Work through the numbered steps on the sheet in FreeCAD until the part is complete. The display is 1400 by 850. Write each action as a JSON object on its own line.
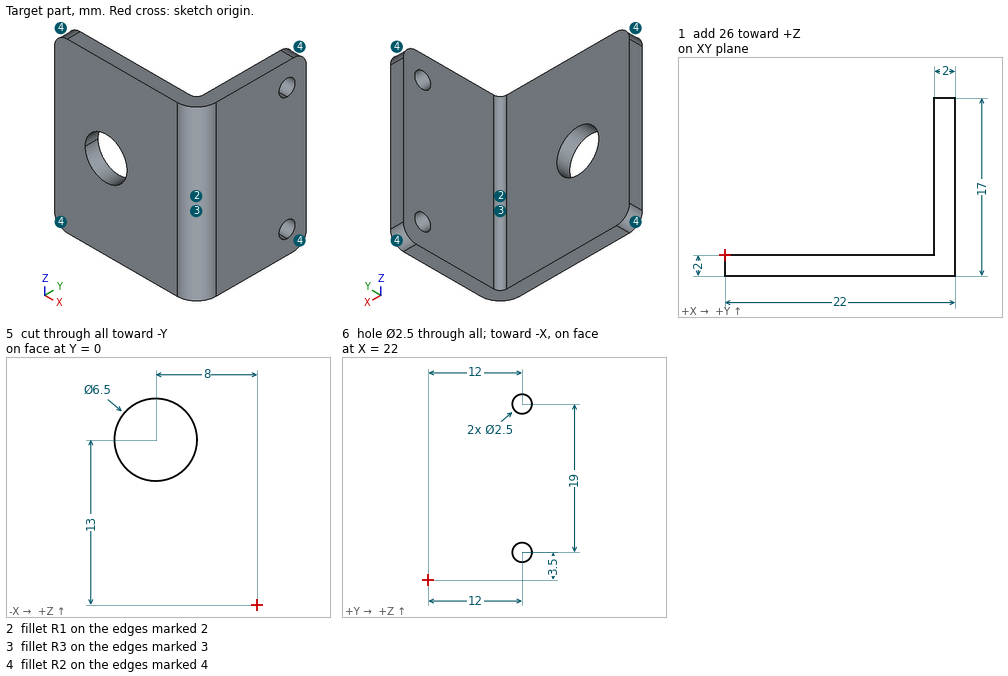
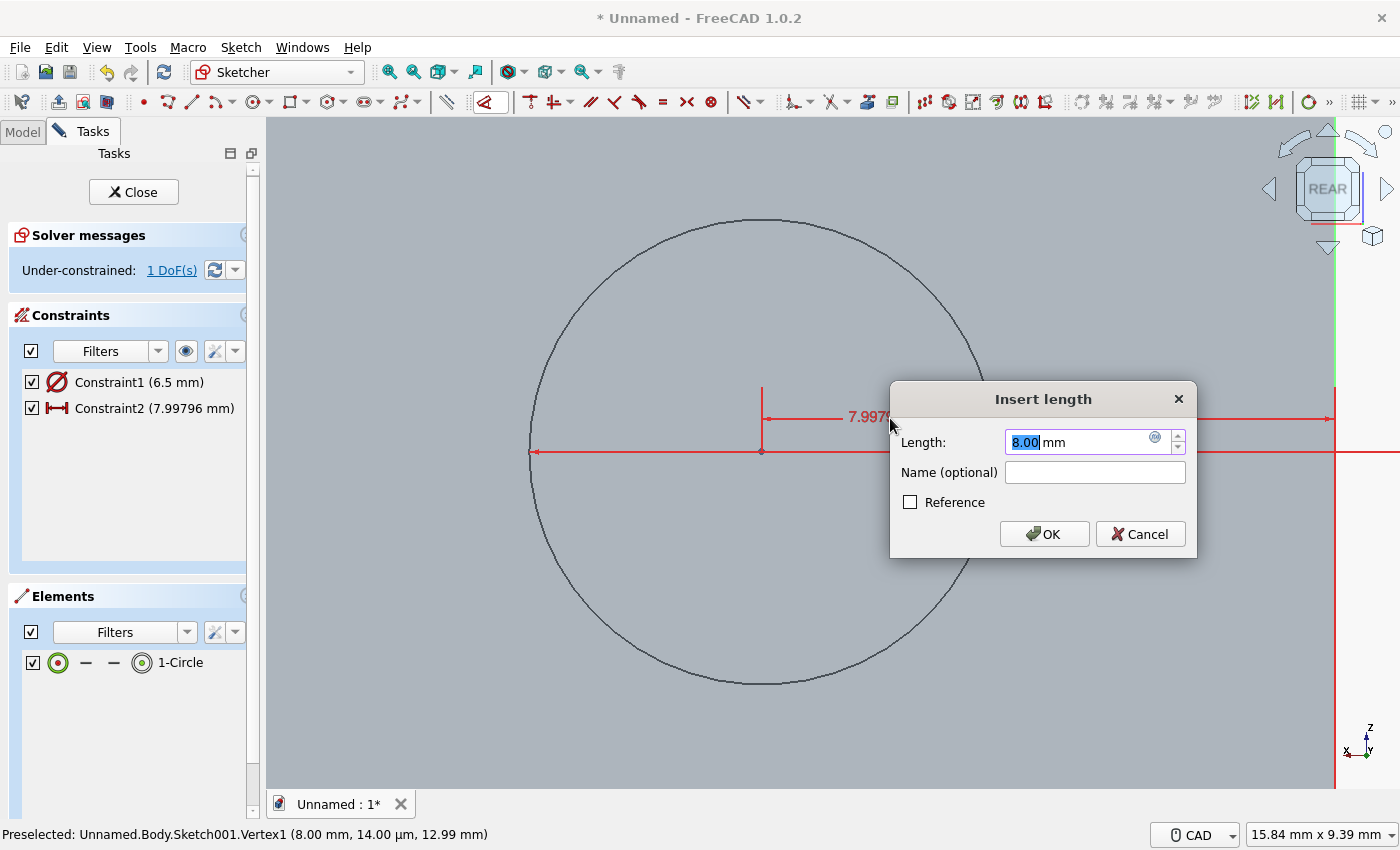
{"action": "type", "text": "8"}
{"action": "key", "text": "Return"}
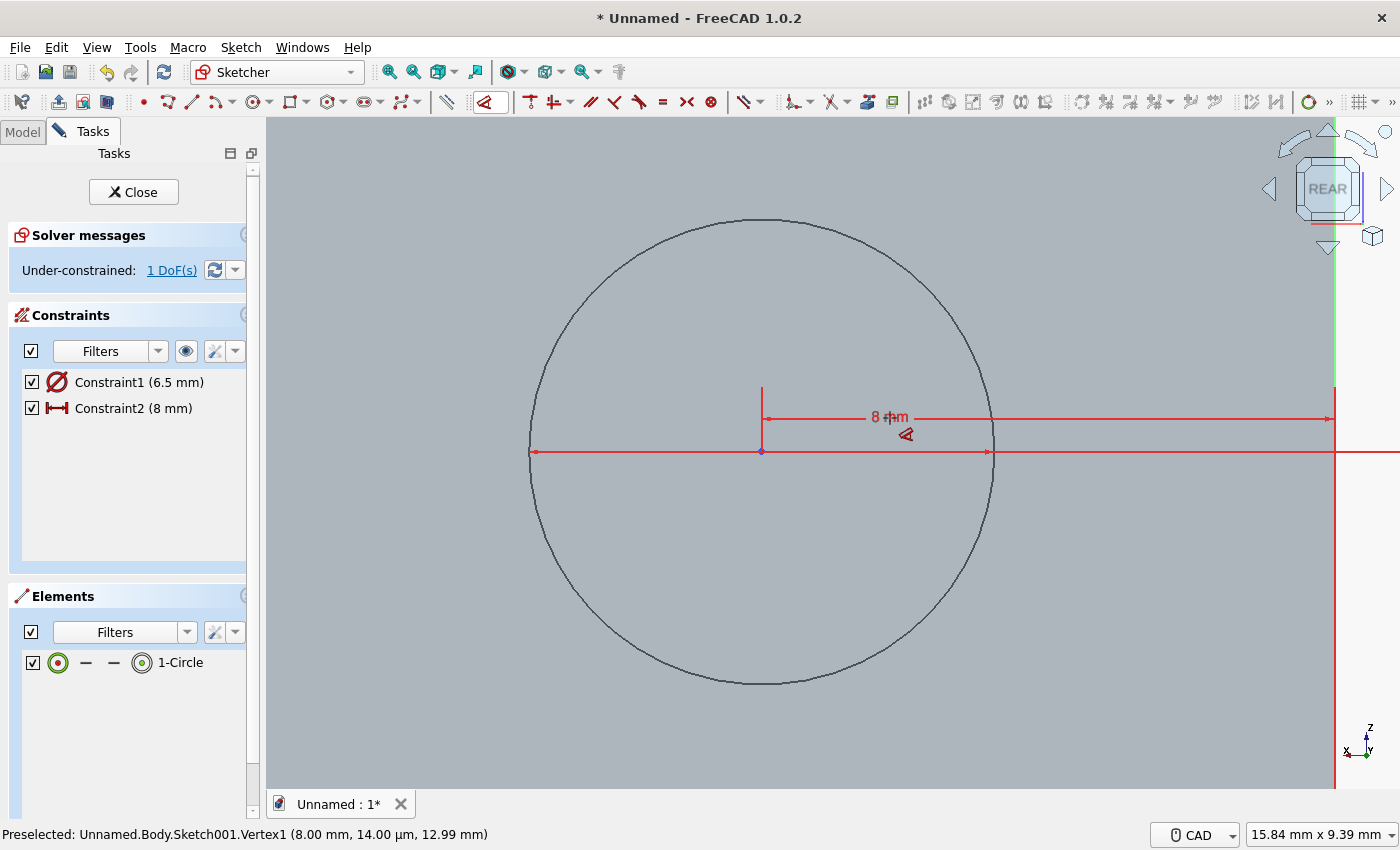
{"action": "left_click", "coordinate": [762, 452]}
{"action": "left_click", "coordinate": [728, 606]}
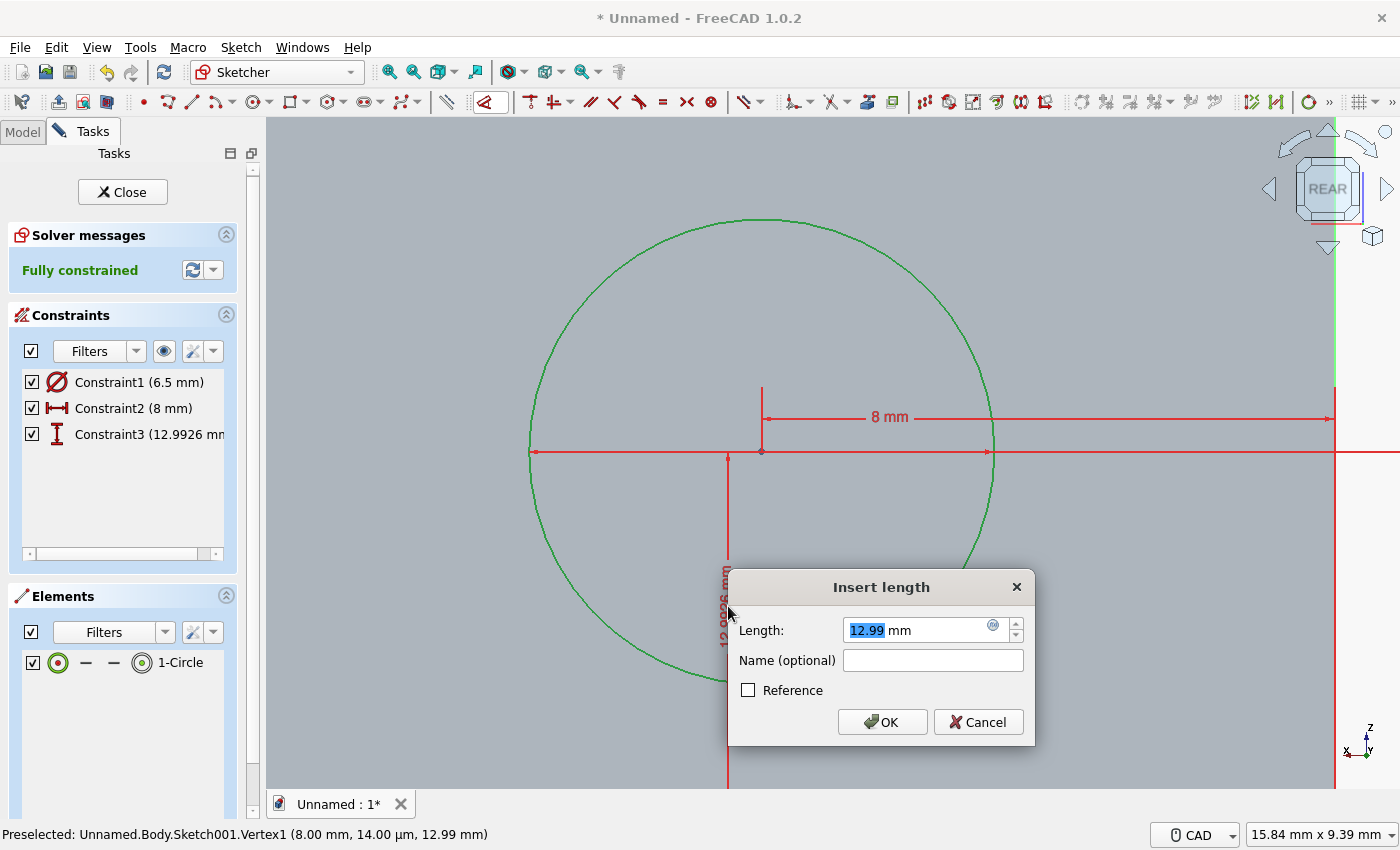
{"action": "type", "text": "13"}
{"action": "key", "text": "Return"}
{"action": "key", "text": "Escape"}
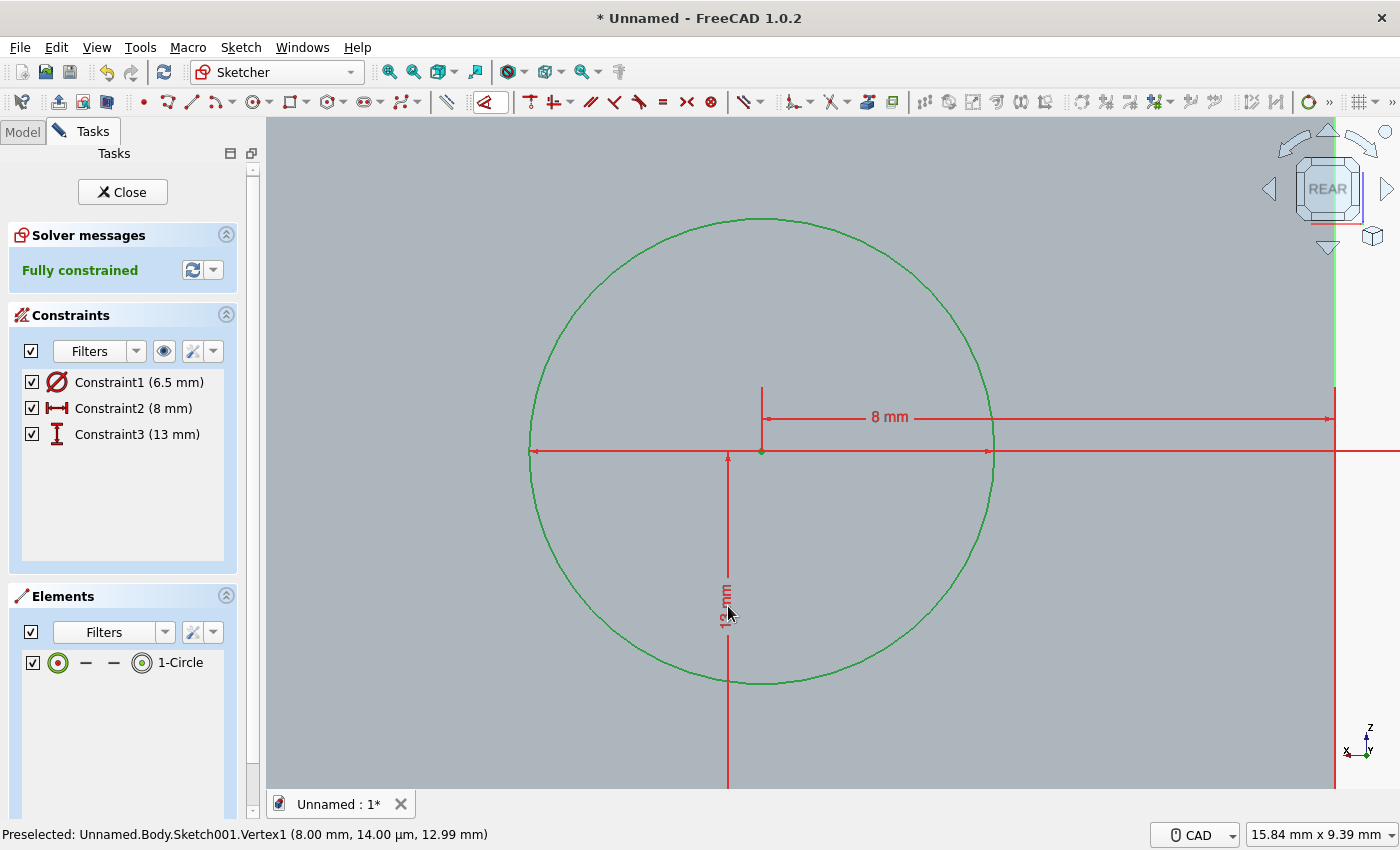
{"action": "left_click", "coordinate": [123, 192]}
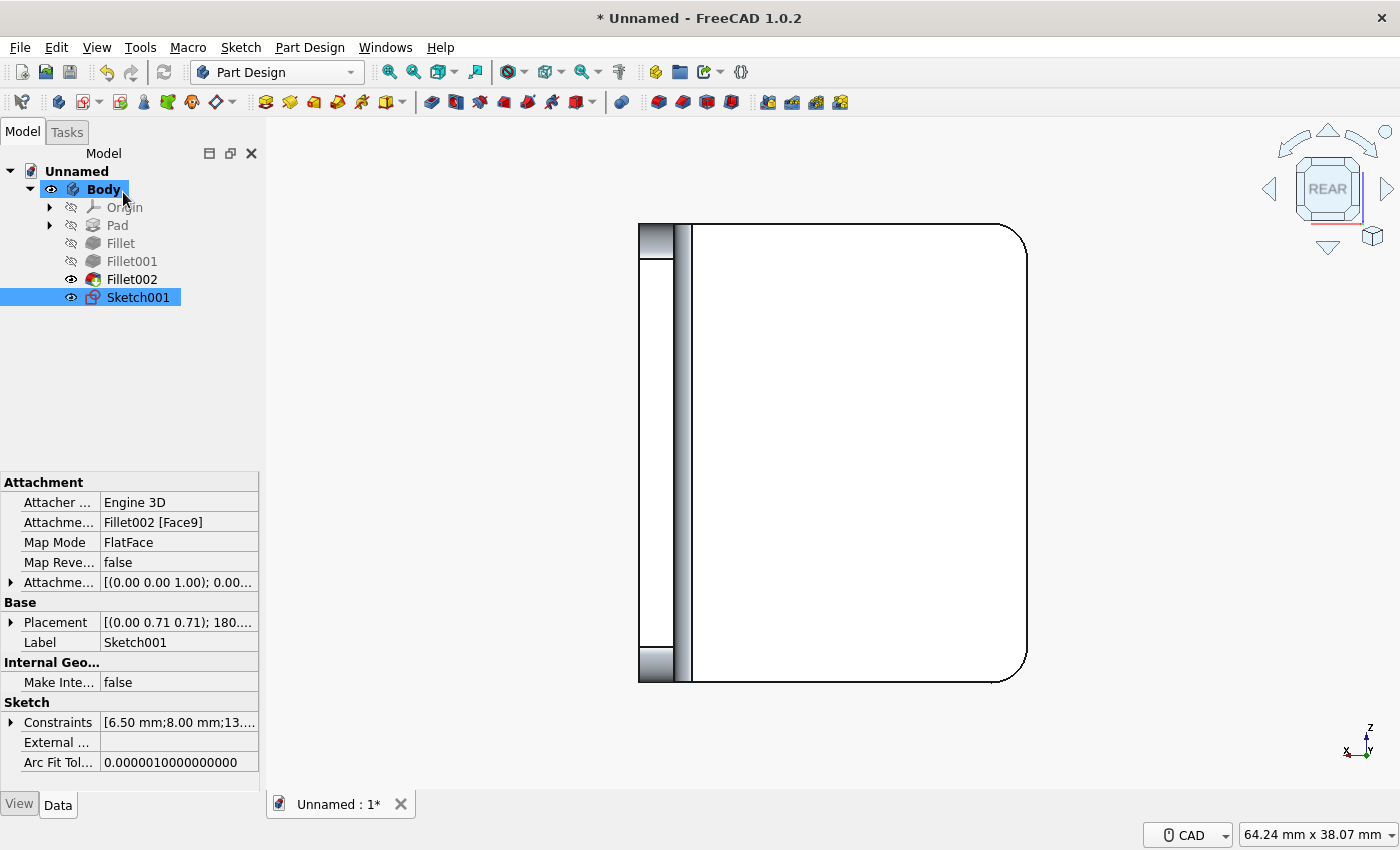
{"action": "left_click", "coordinate": [432, 102]}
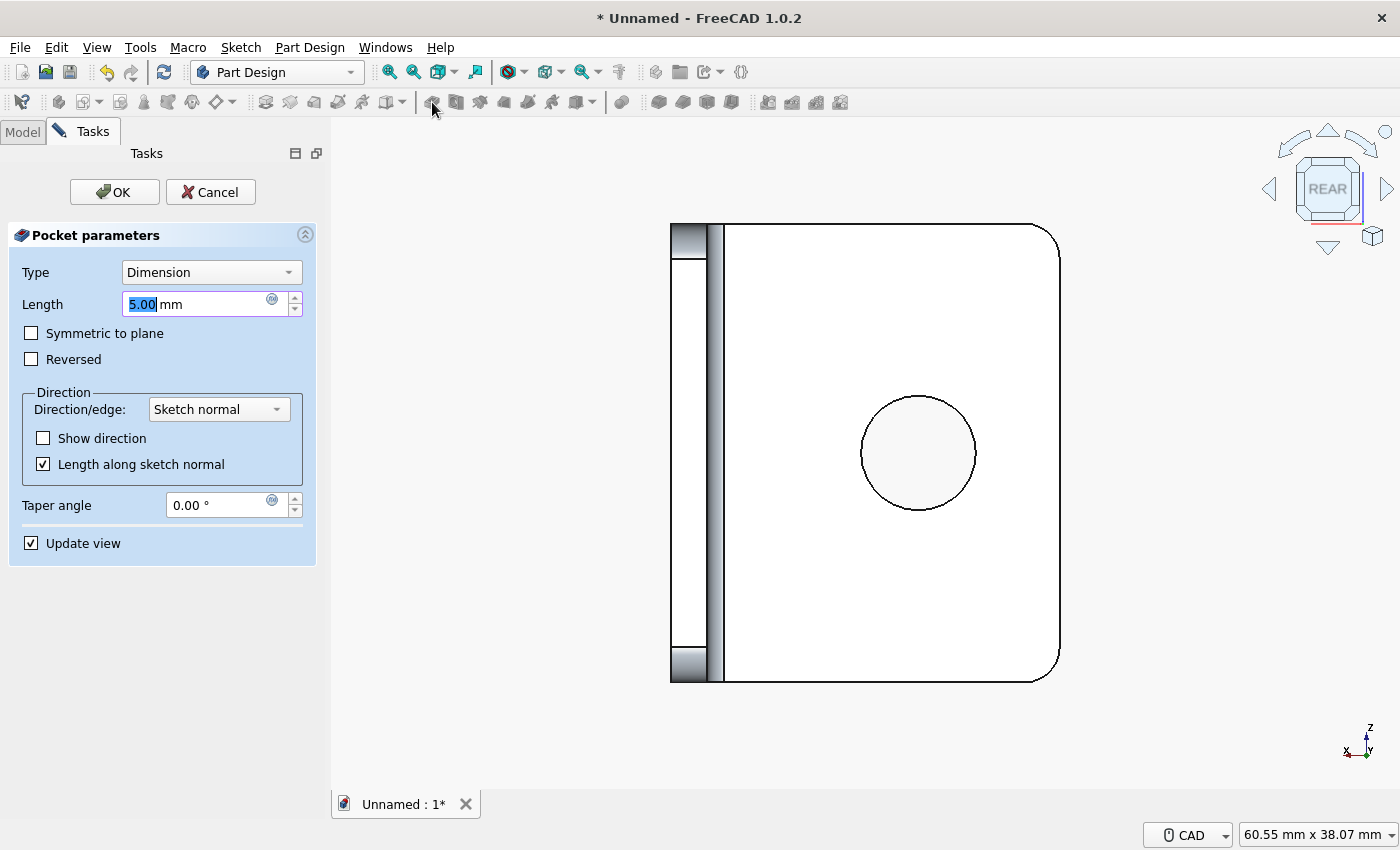
{"action": "left_click", "coordinate": [212, 272]}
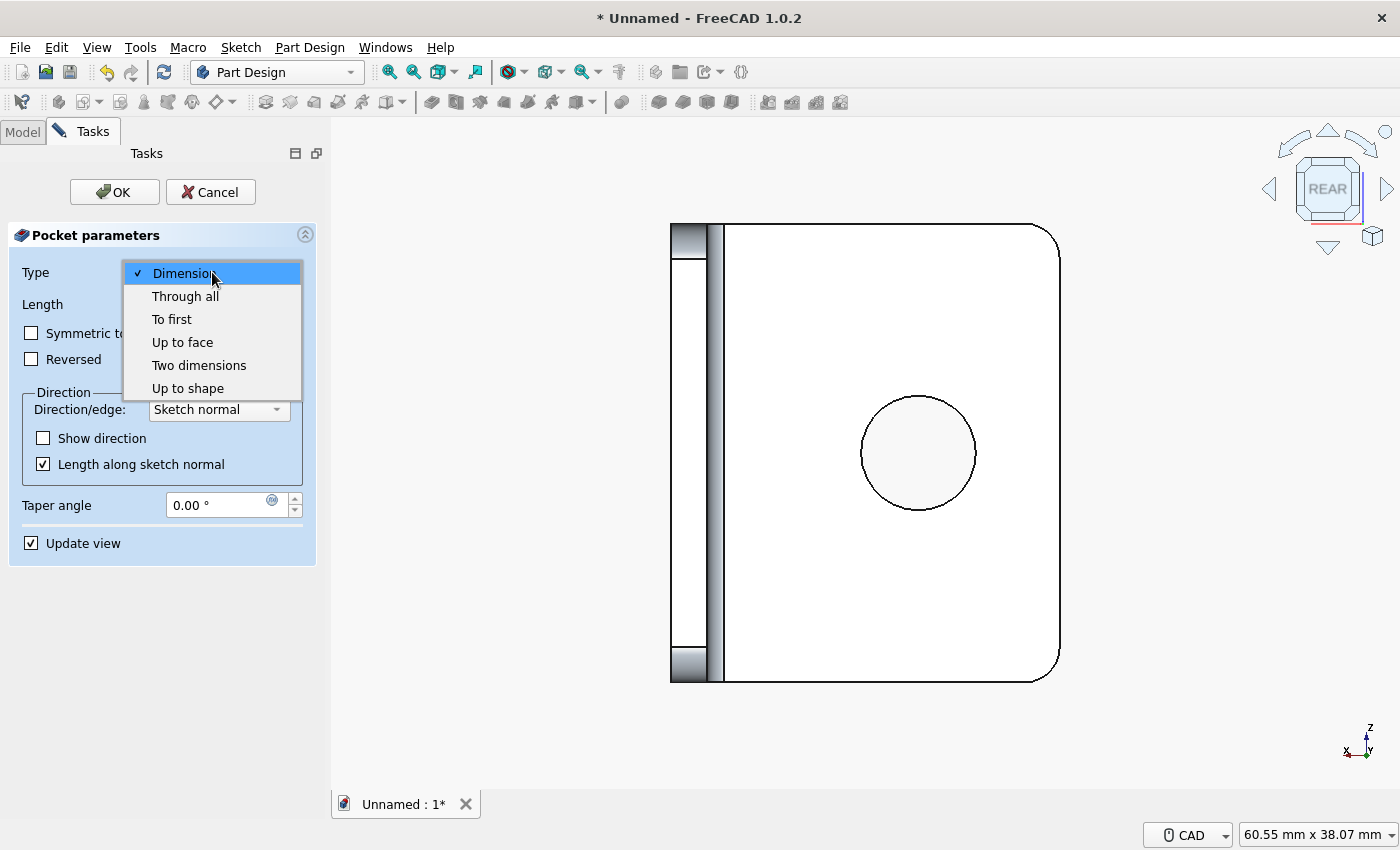
{"action": "left_click", "coordinate": [212, 296]}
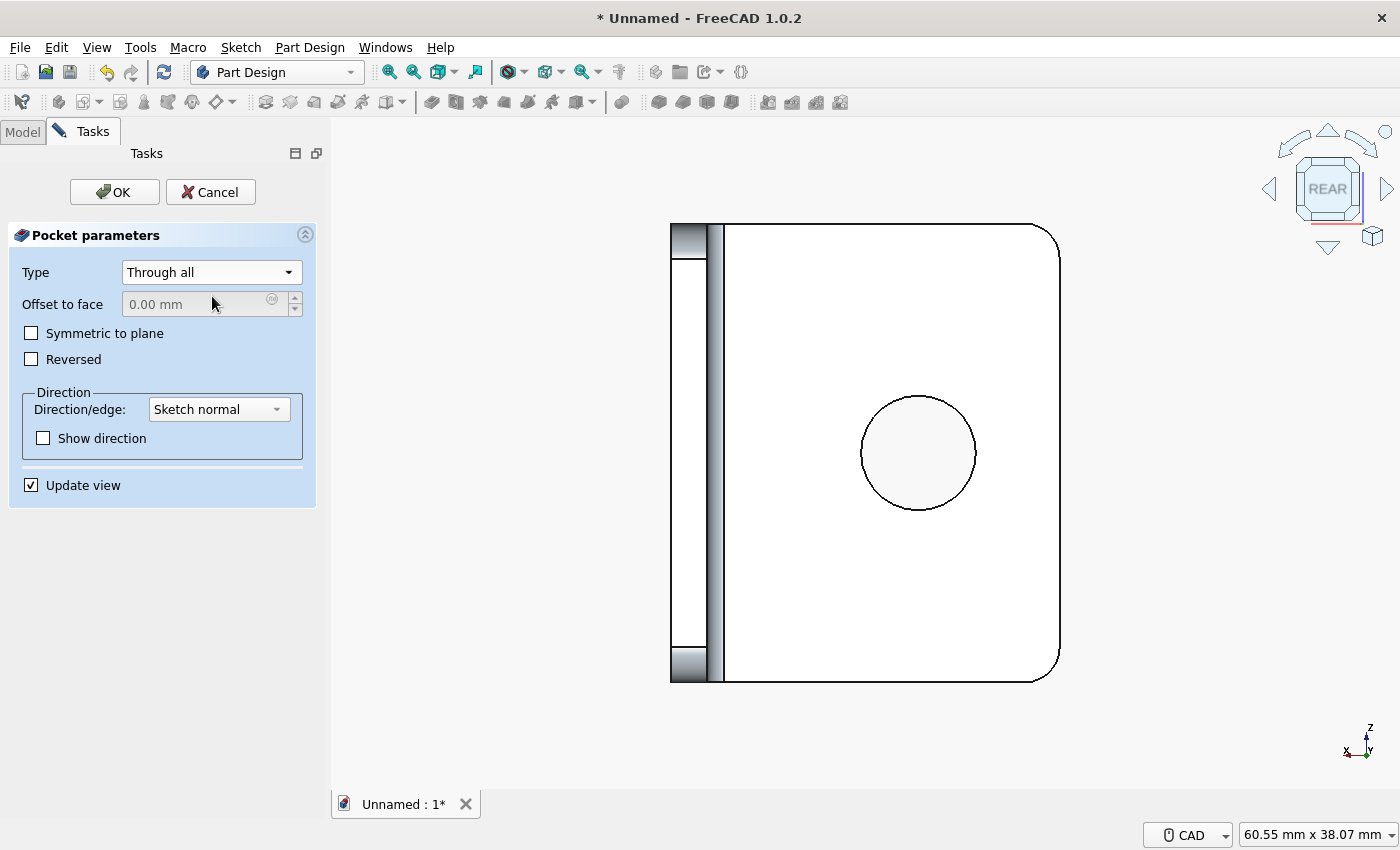
{"action": "left_click", "coordinate": [115, 192]}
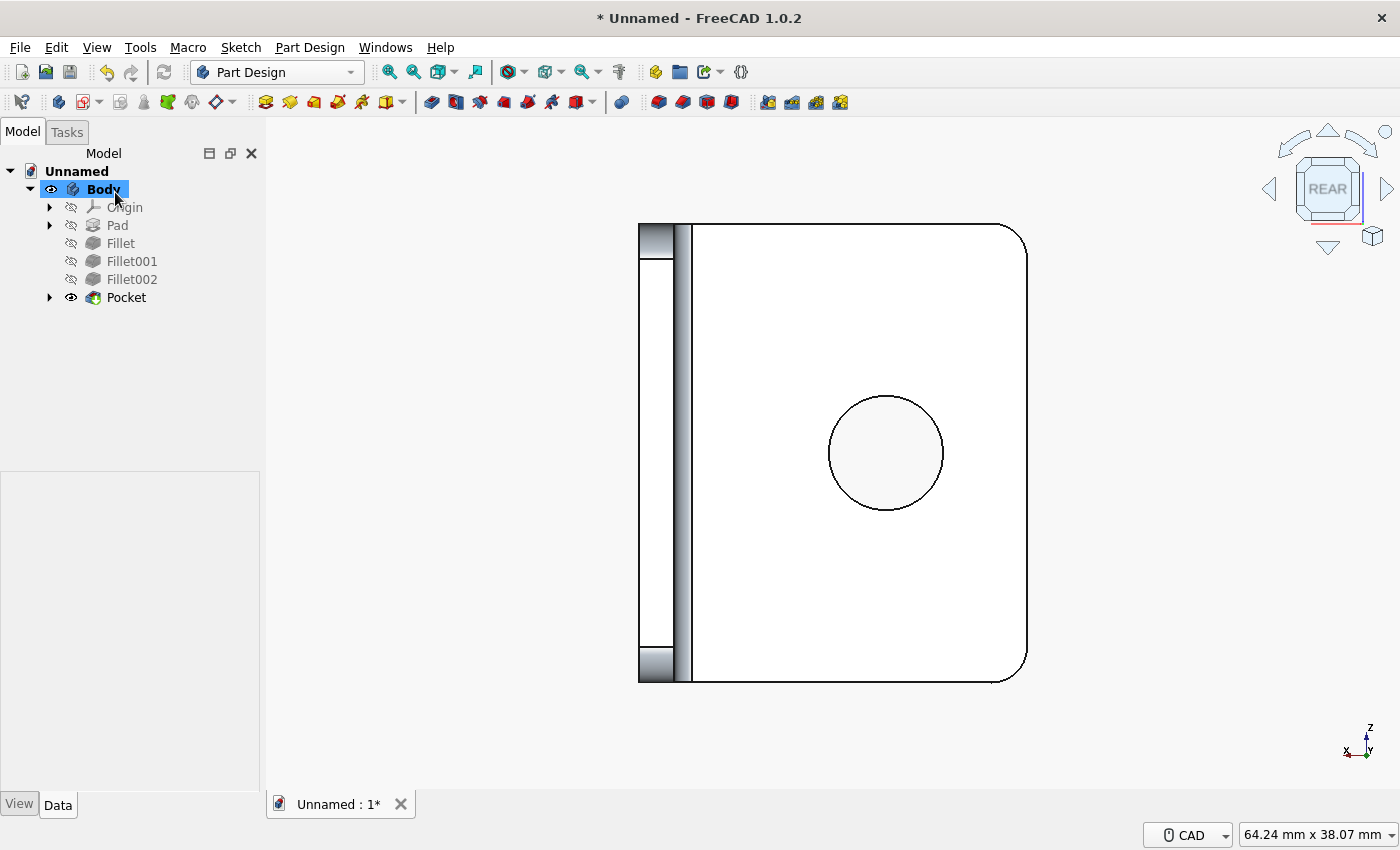
{"action": "key", "text": "0"}